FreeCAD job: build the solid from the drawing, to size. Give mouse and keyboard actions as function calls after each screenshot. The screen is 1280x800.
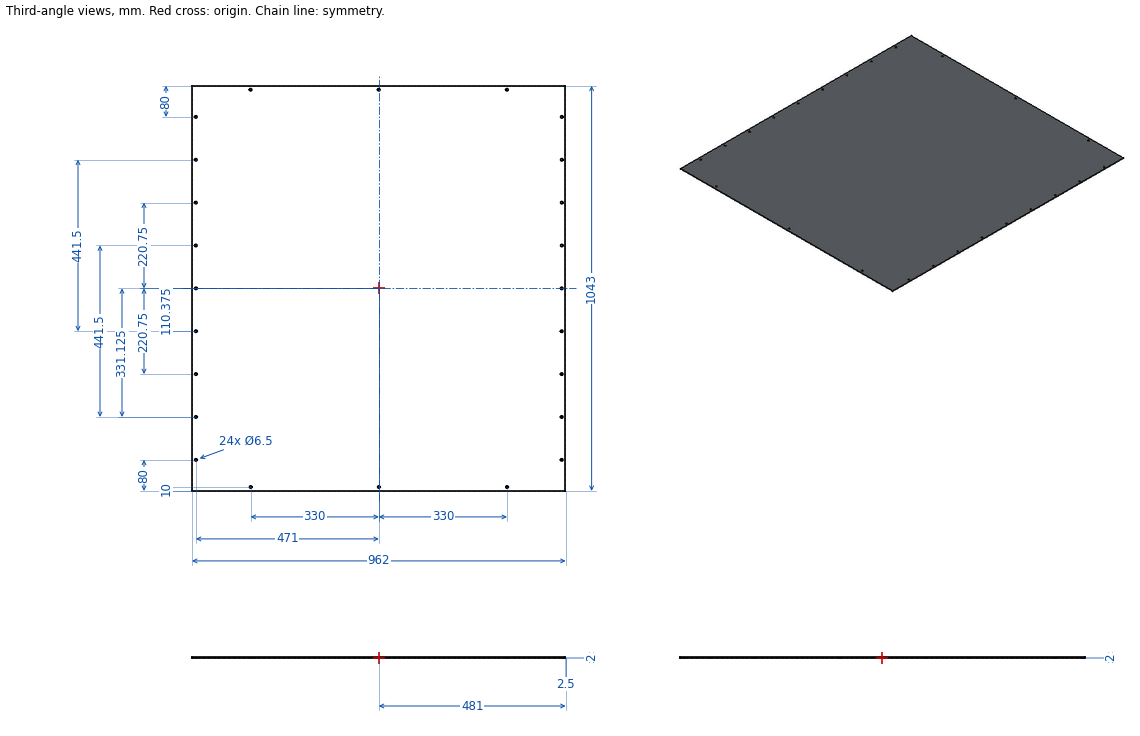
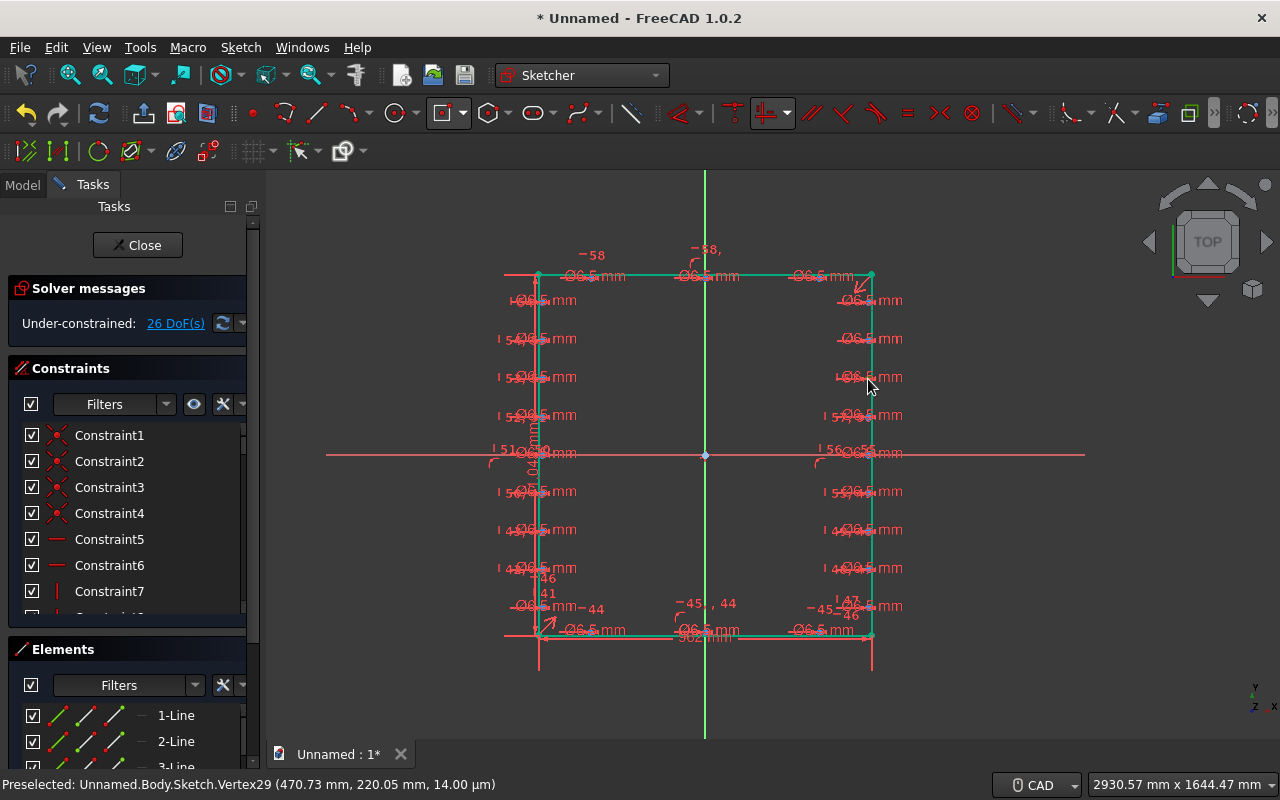
click(868, 341)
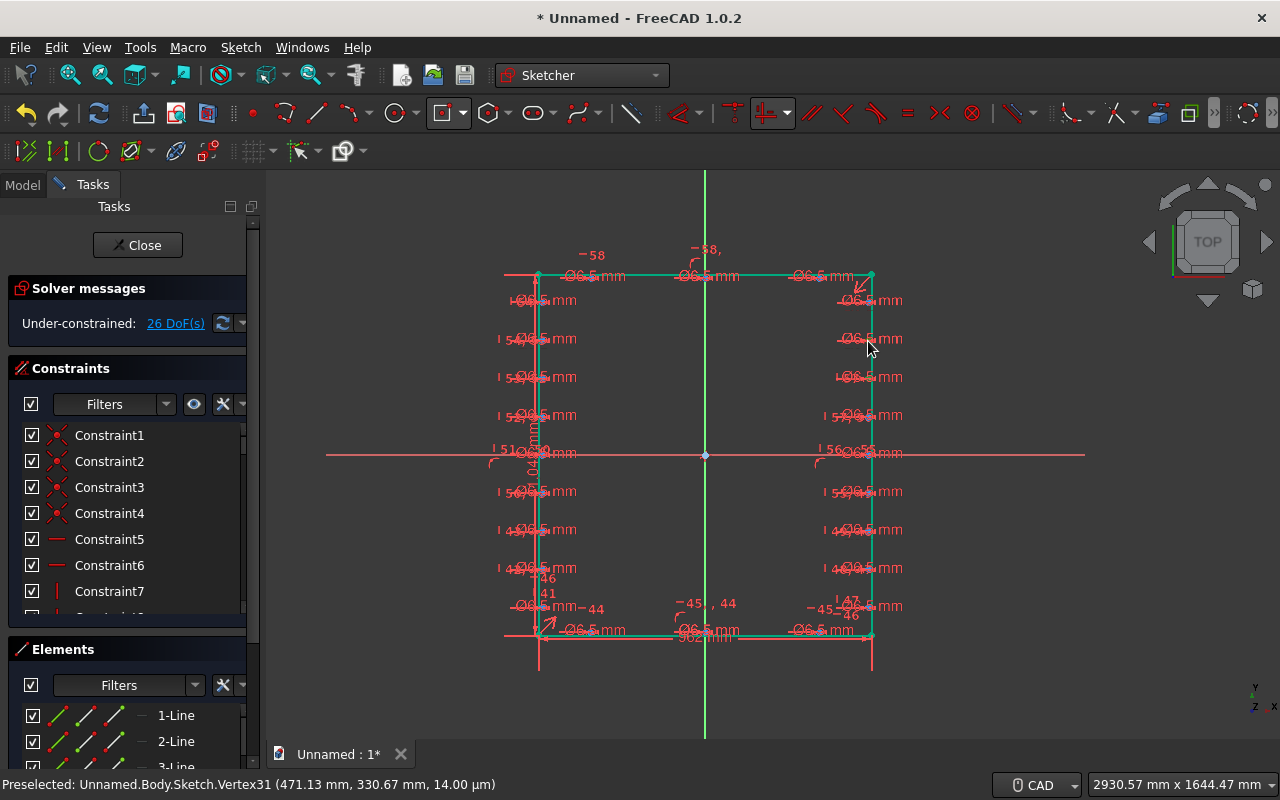
click(790, 114)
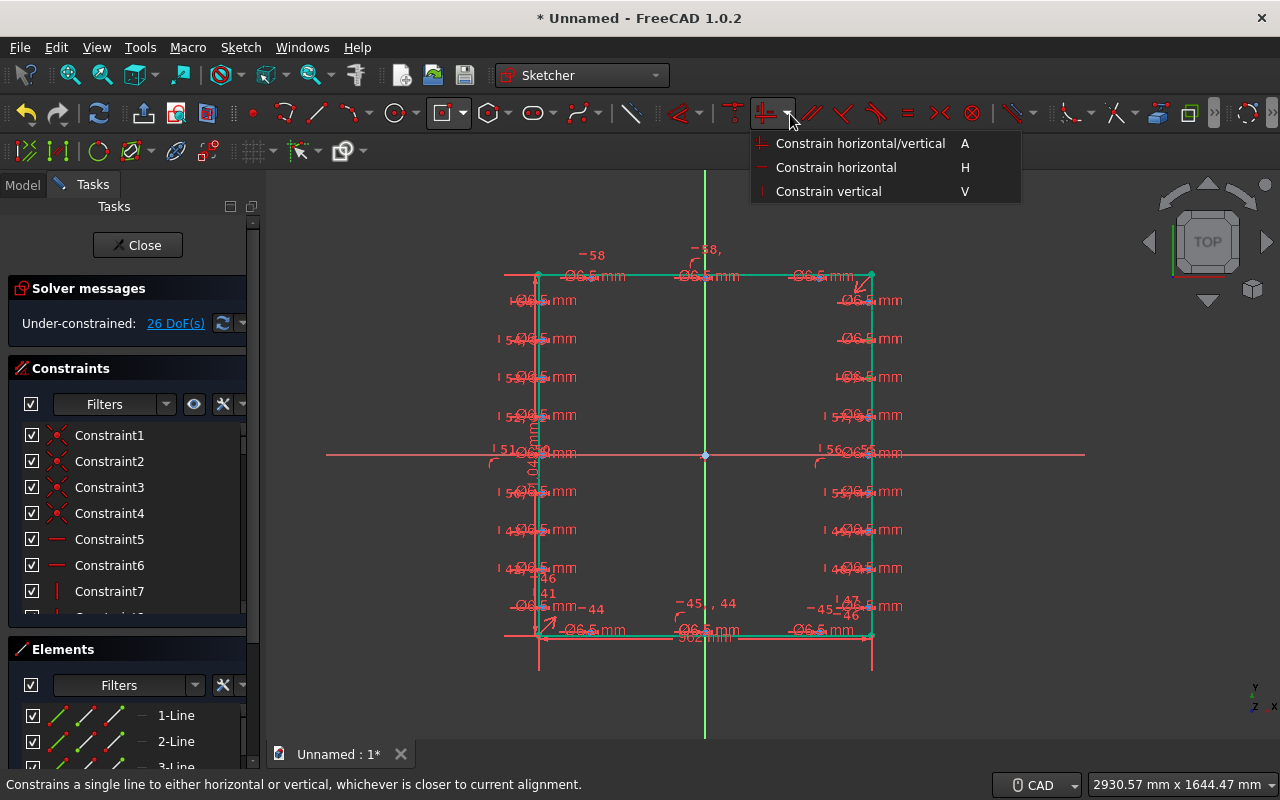
click(886, 191)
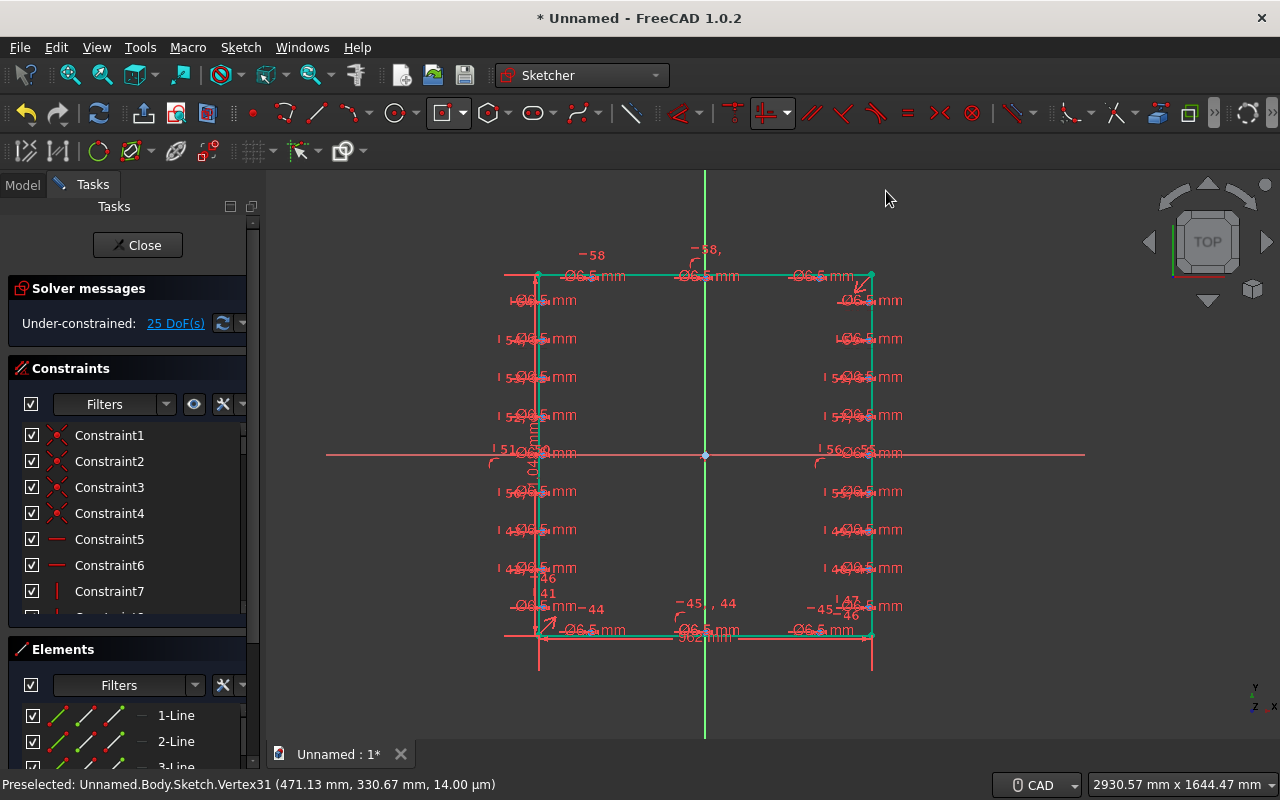
click(705, 278)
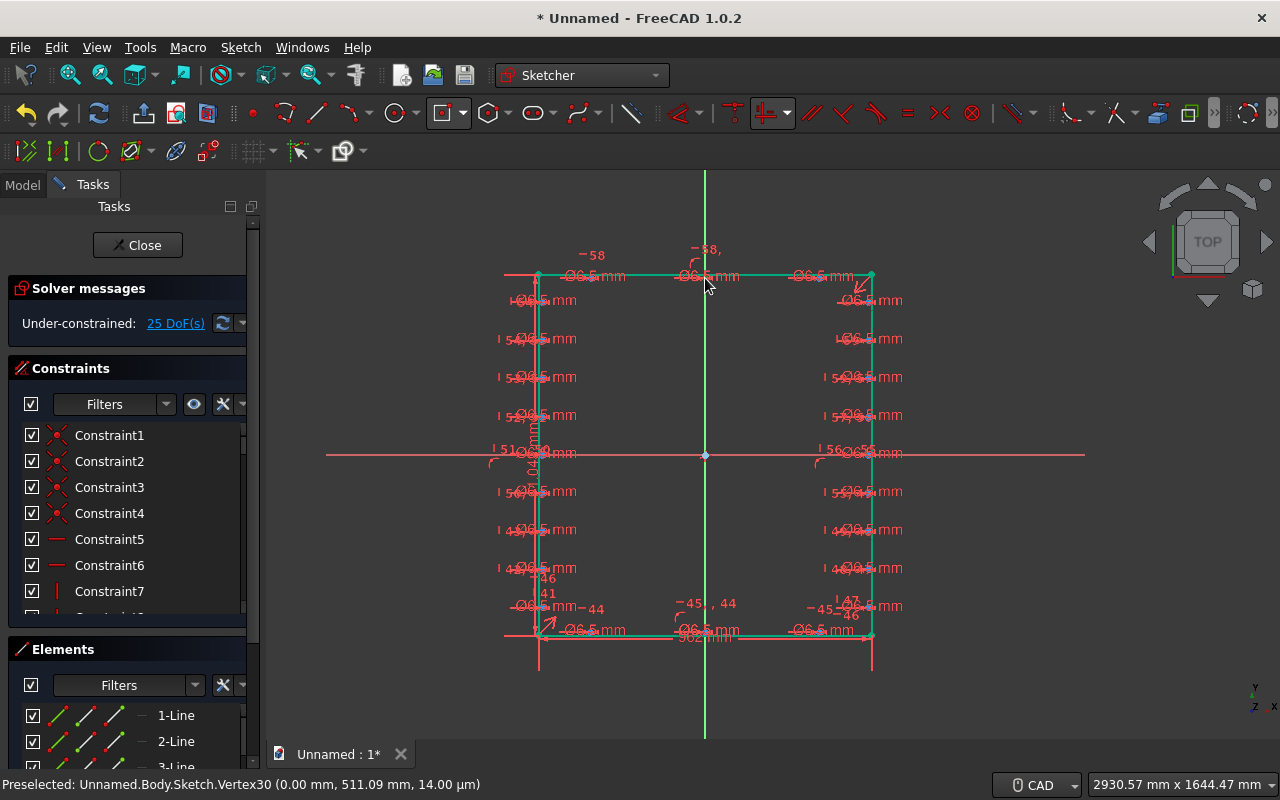
click(819, 278)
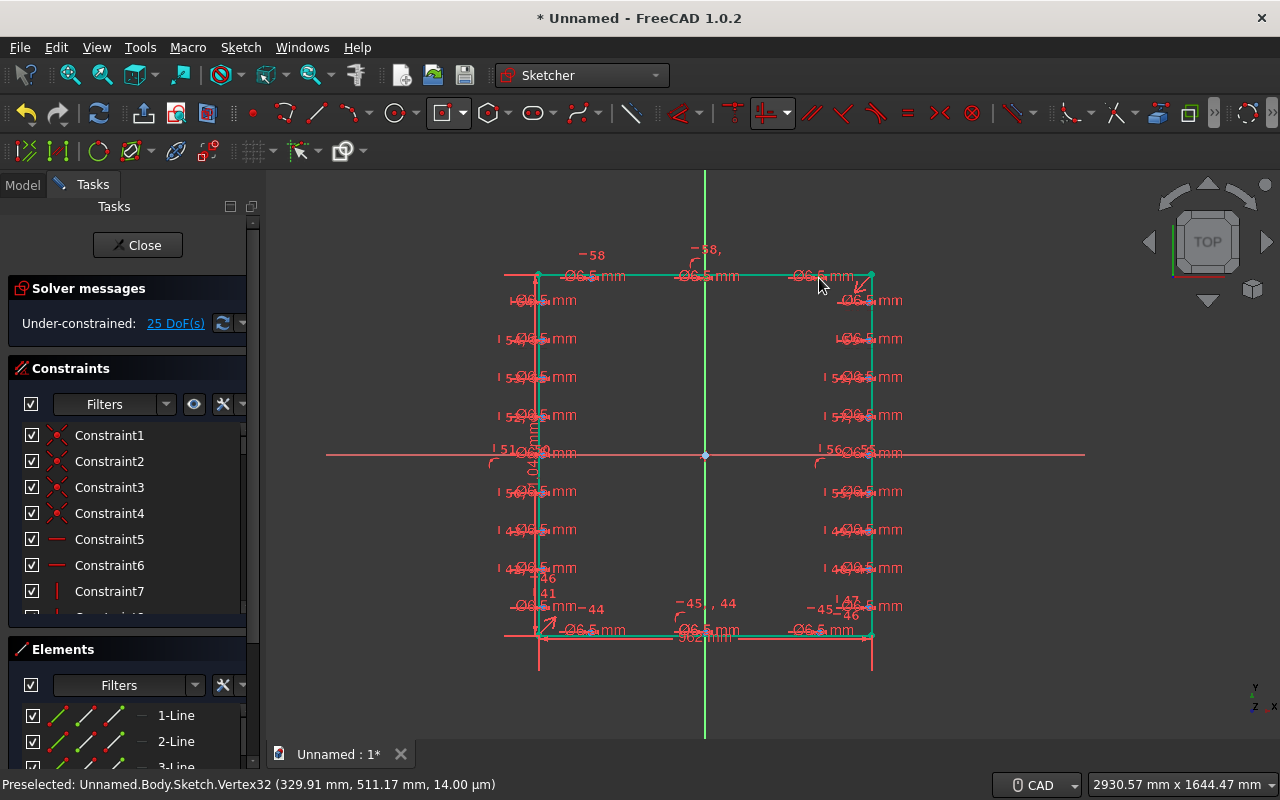
key(h)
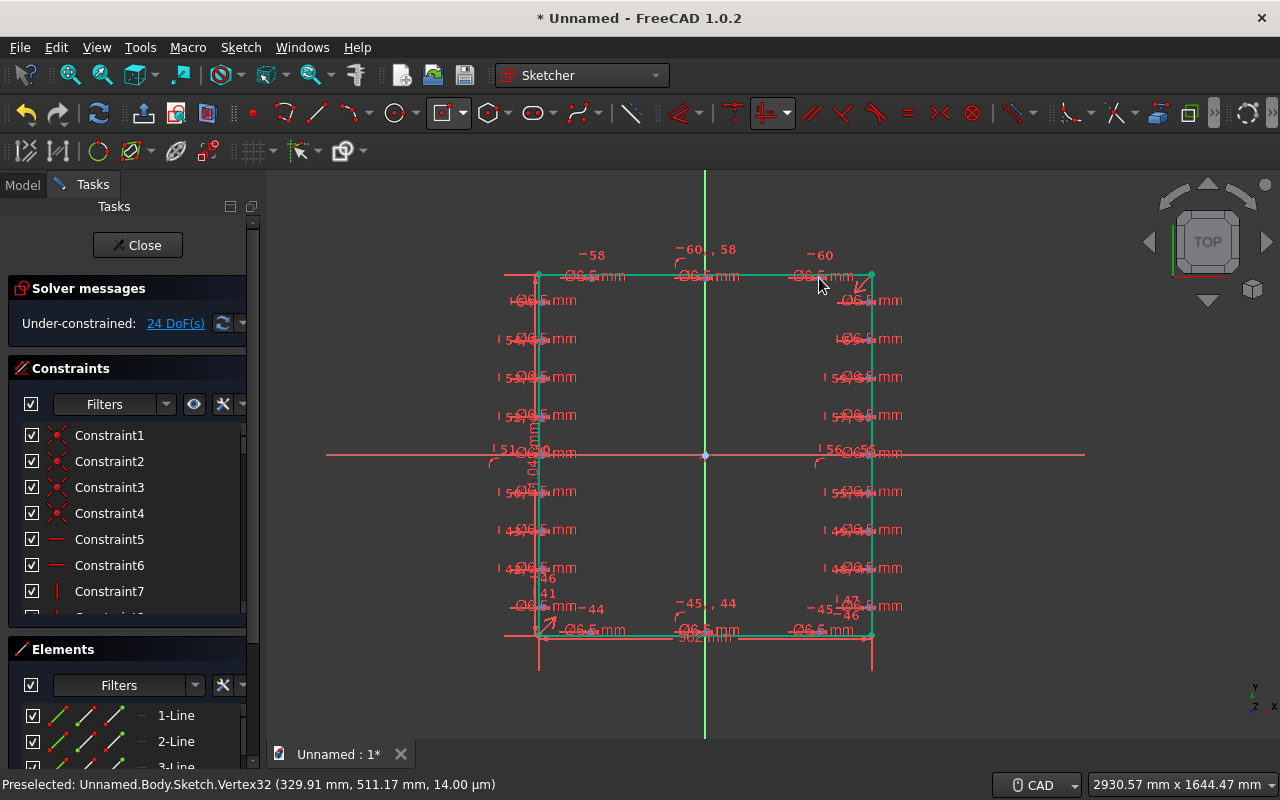
click(868, 341)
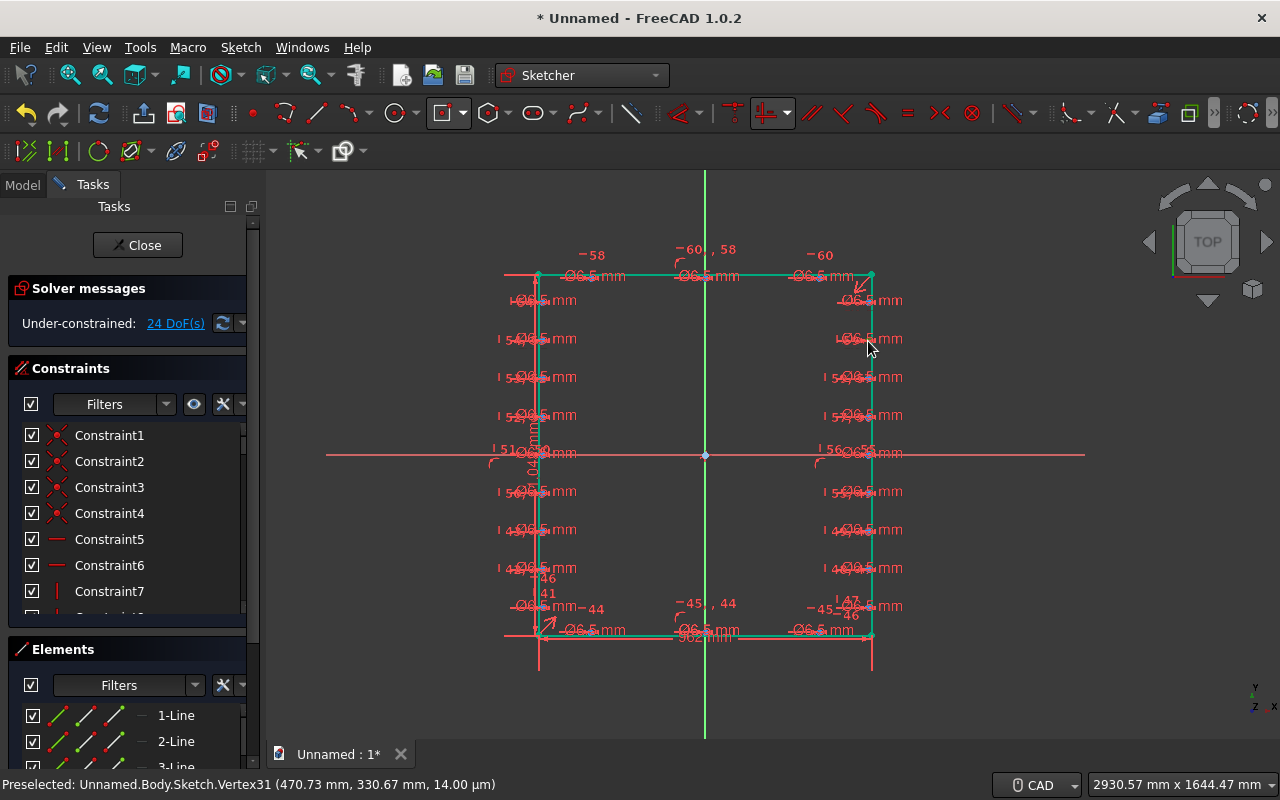
click(868, 303)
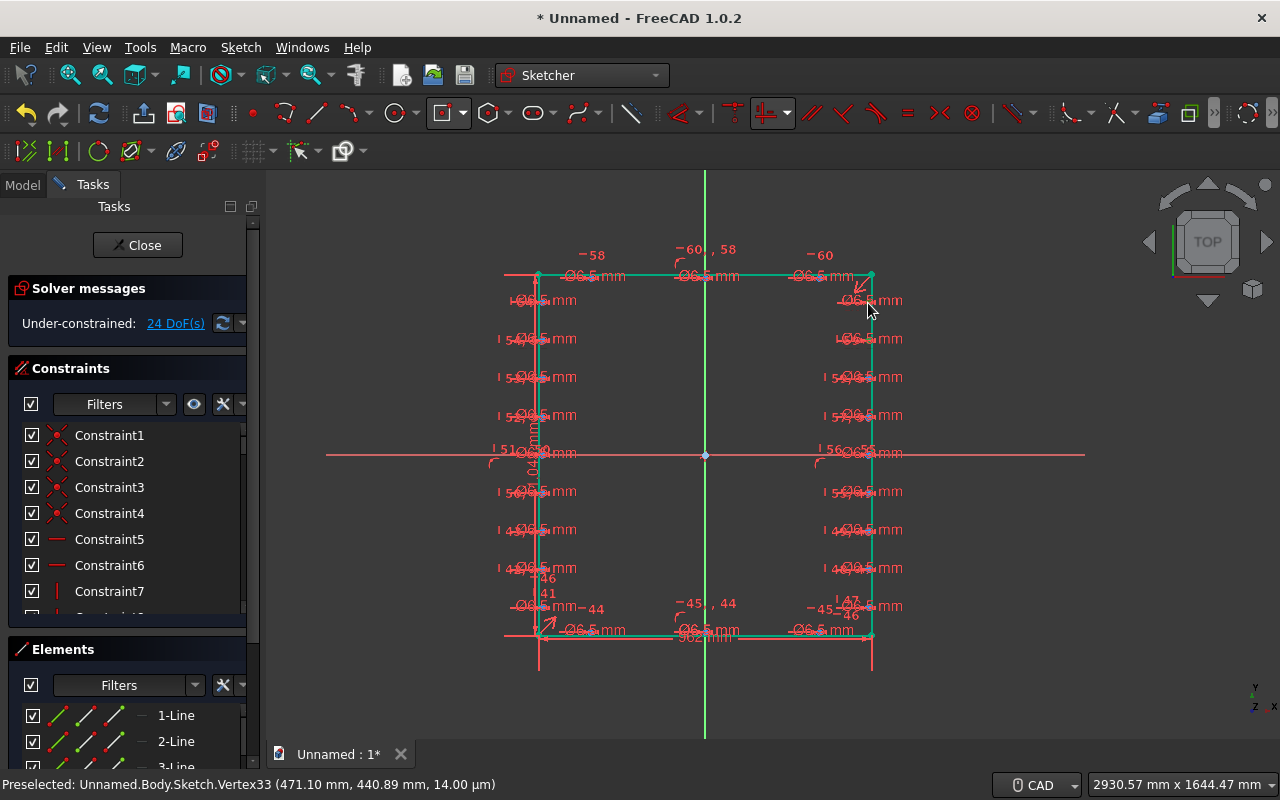
click(790, 114)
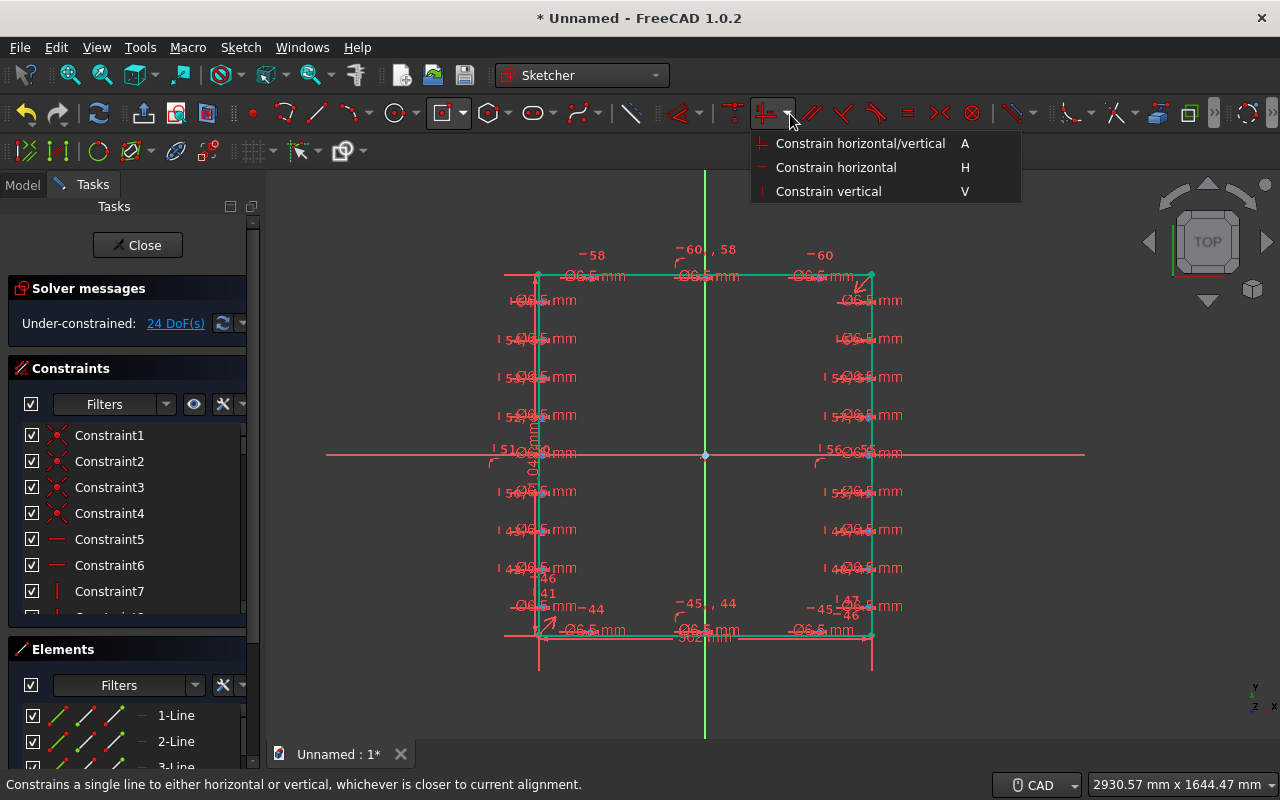
click(886, 191)